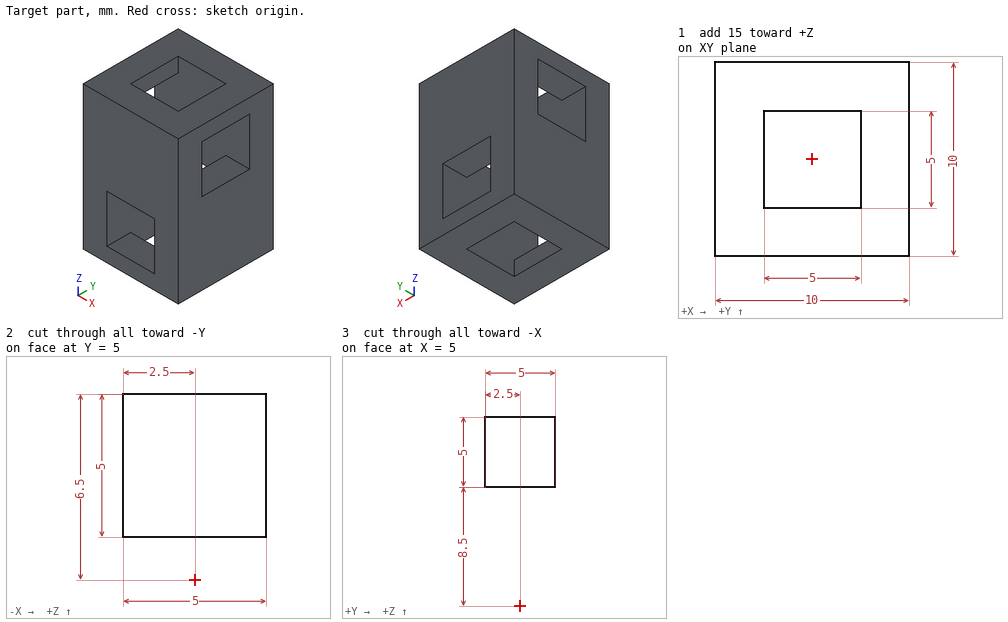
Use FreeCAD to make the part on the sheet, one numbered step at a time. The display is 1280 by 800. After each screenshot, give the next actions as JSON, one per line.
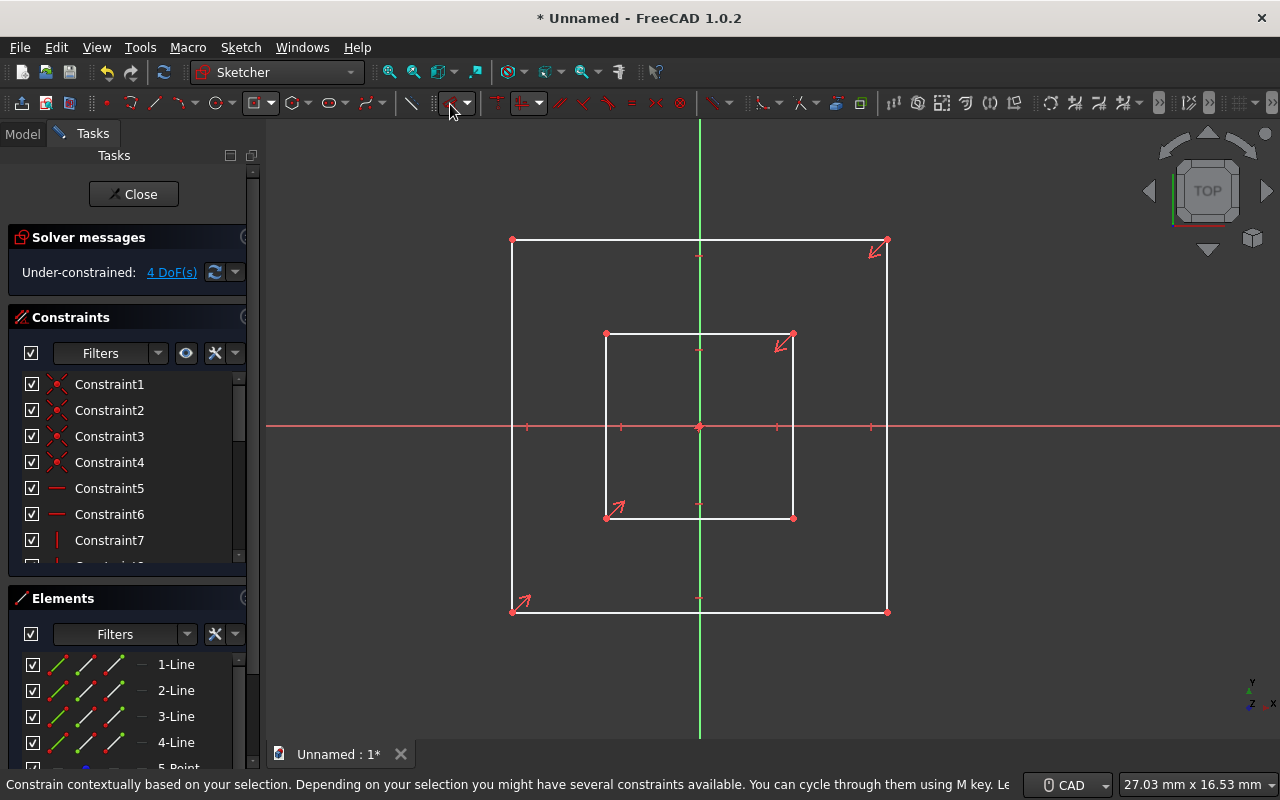
{"action": "left_click", "coordinate": [662, 519]}
{"action": "left_click", "coordinate": [657, 553]}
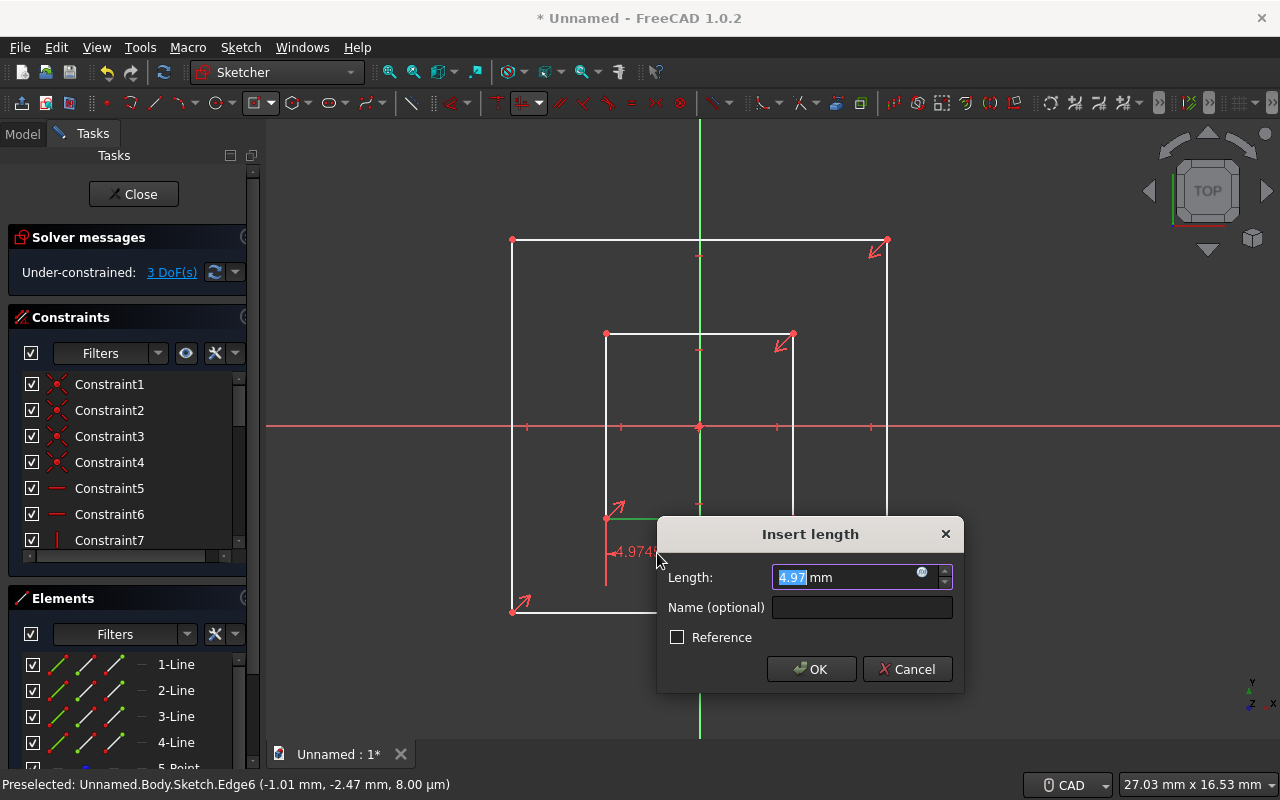
{"action": "type", "text": "5"}
{"action": "key", "text": "Return"}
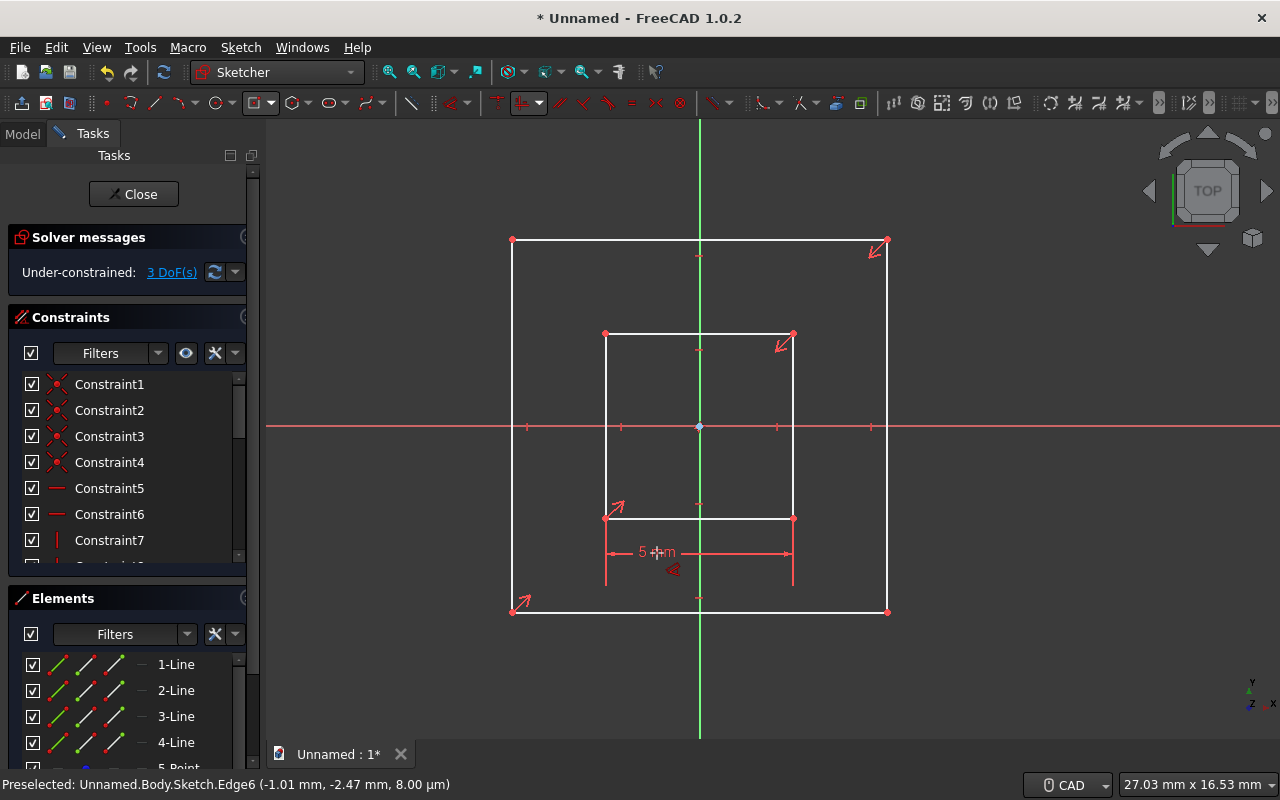
{"action": "left_click", "coordinate": [793, 463]}
{"action": "left_click", "coordinate": [827, 384]}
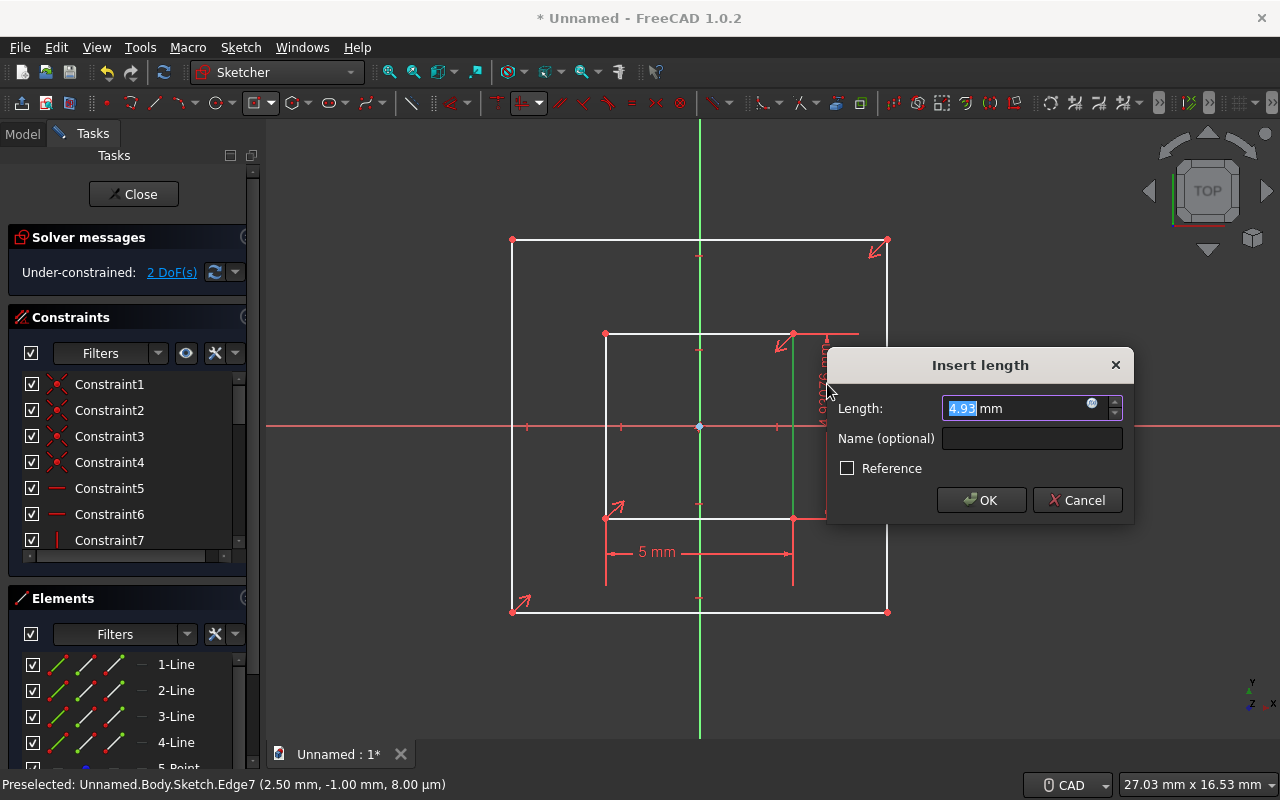
{"action": "type", "text": "5"}
{"action": "key", "text": "Return"}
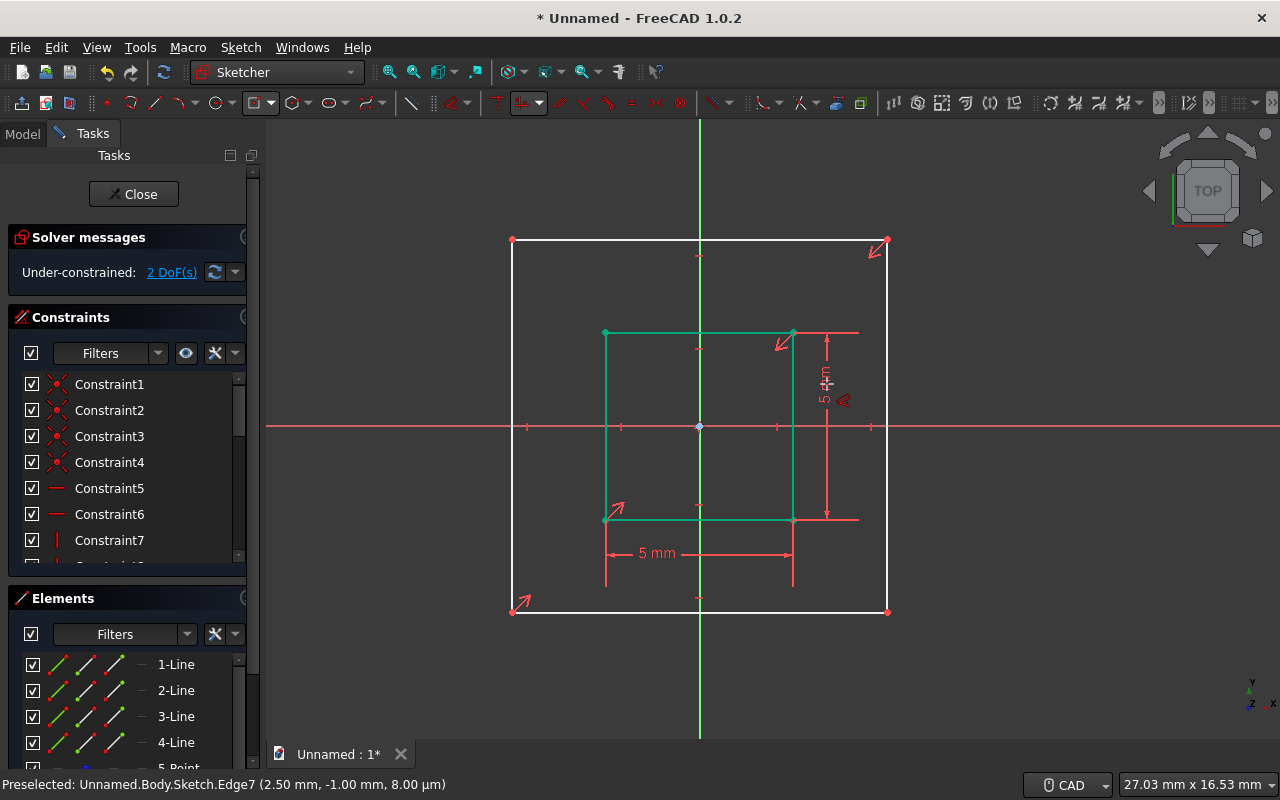
{"action": "left_click", "coordinate": [625, 613]}
{"action": "left_click", "coordinate": [614, 647]}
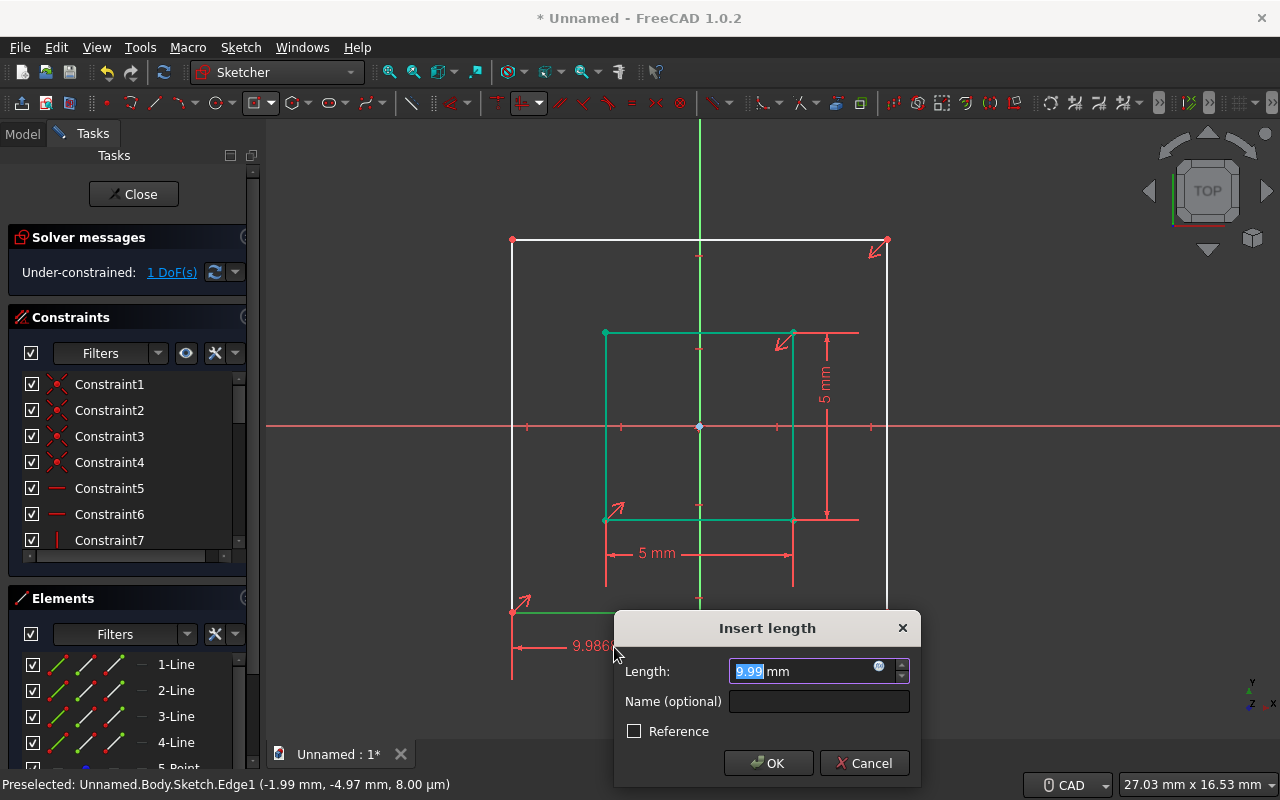
{"action": "type", "text": "10"}
{"action": "key", "text": "Return"}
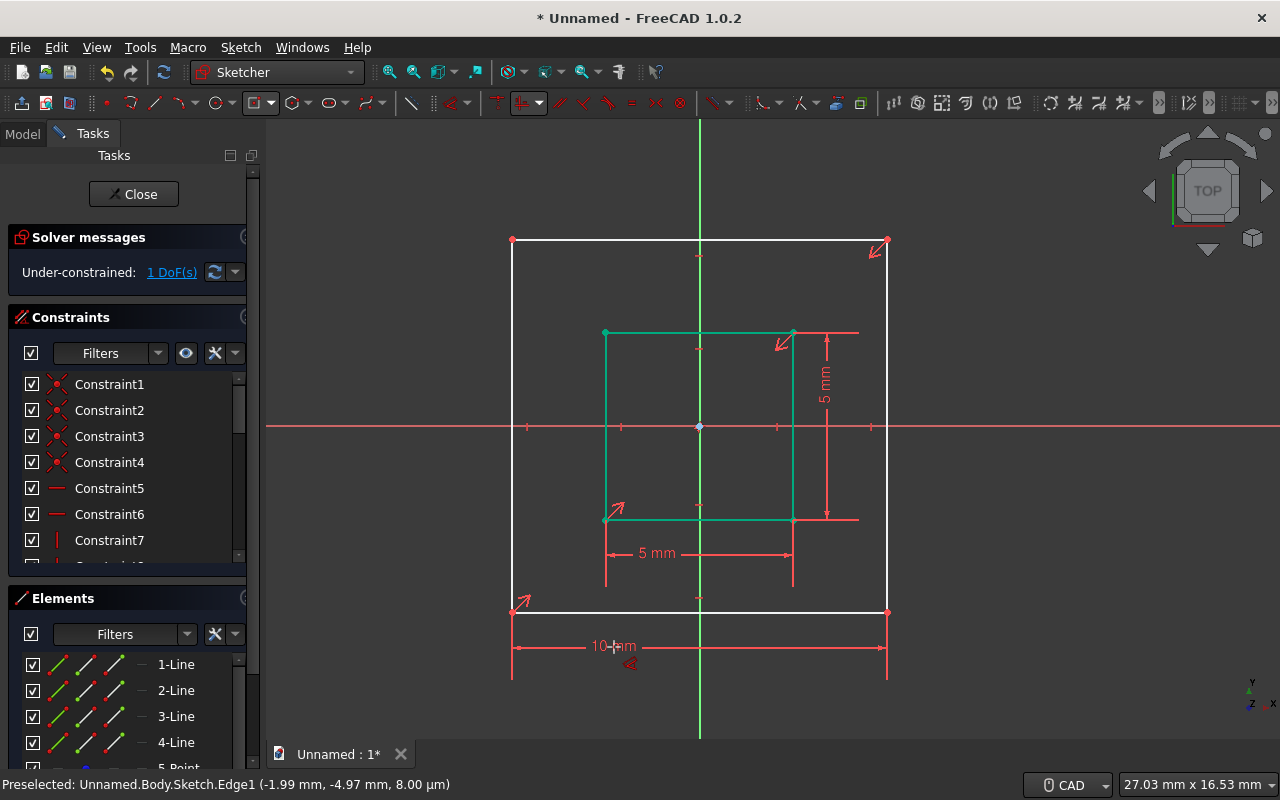
{"action": "left_click", "coordinate": [887, 501]}
{"action": "left_click", "coordinate": [921, 341]}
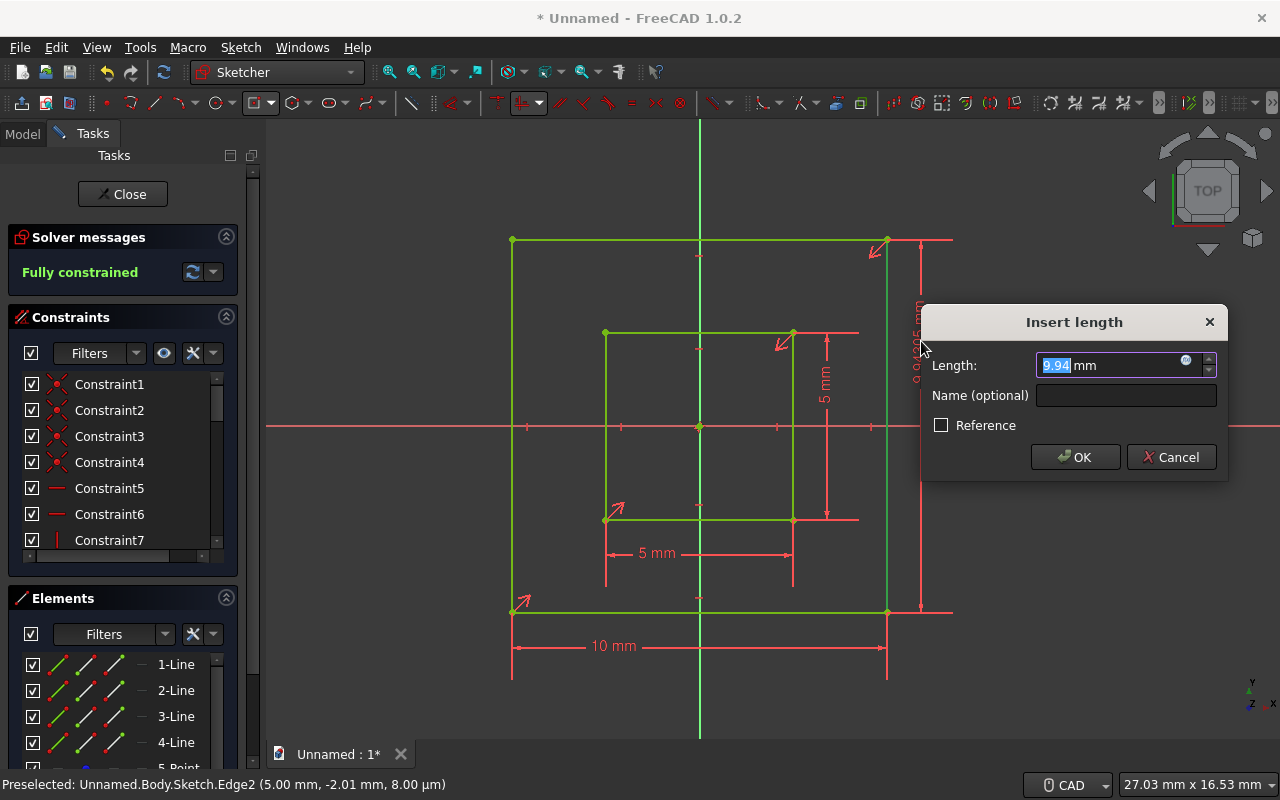
{"action": "type", "text": "10"}
{"action": "key", "text": "Return"}
{"action": "key", "text": "Escape"}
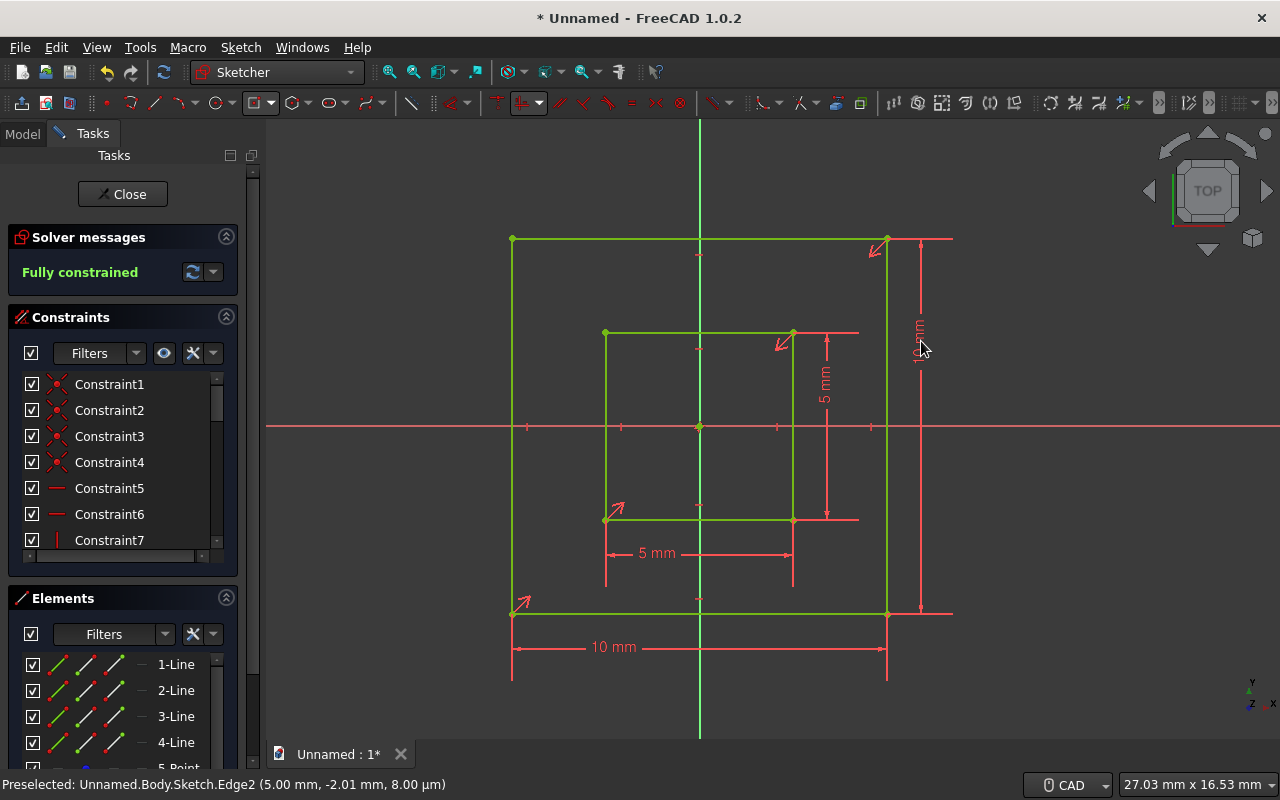
{"action": "left_click", "coordinate": [123, 194]}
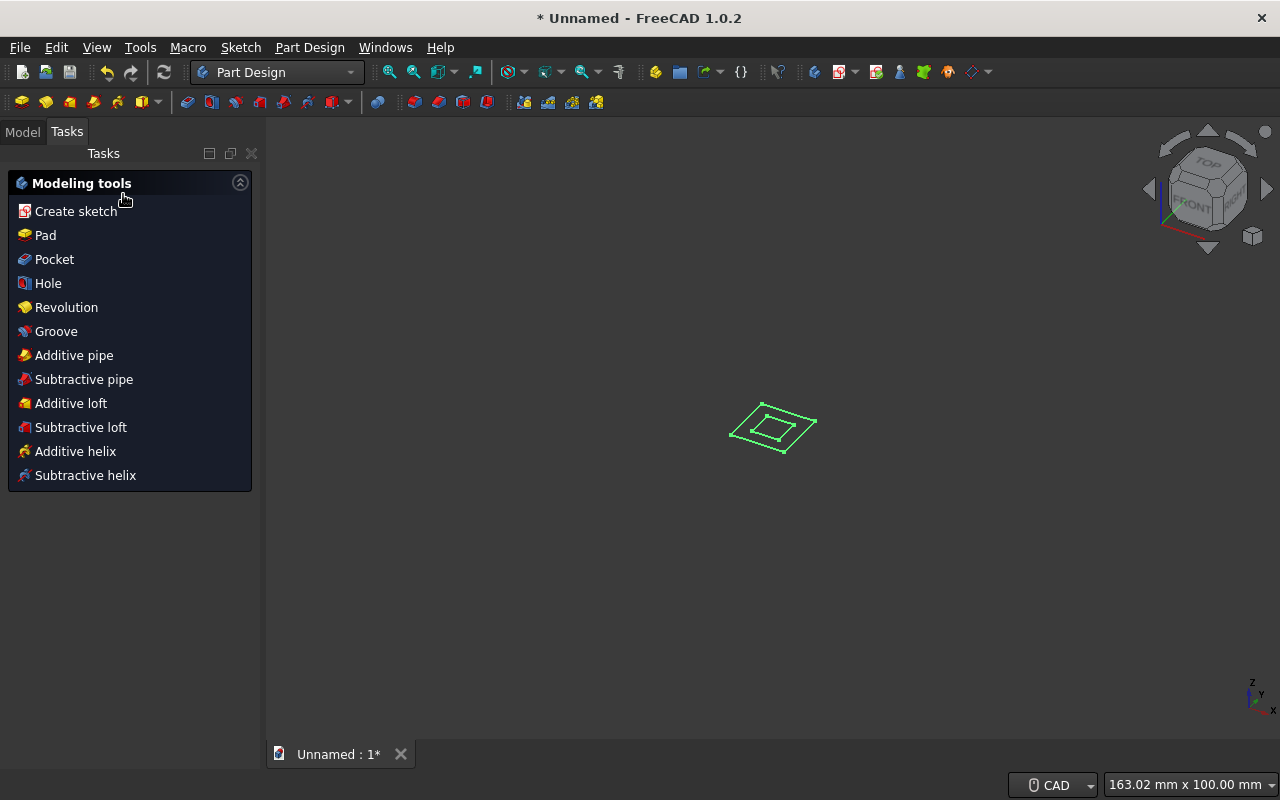
{"action": "left_click", "coordinate": [22, 102]}